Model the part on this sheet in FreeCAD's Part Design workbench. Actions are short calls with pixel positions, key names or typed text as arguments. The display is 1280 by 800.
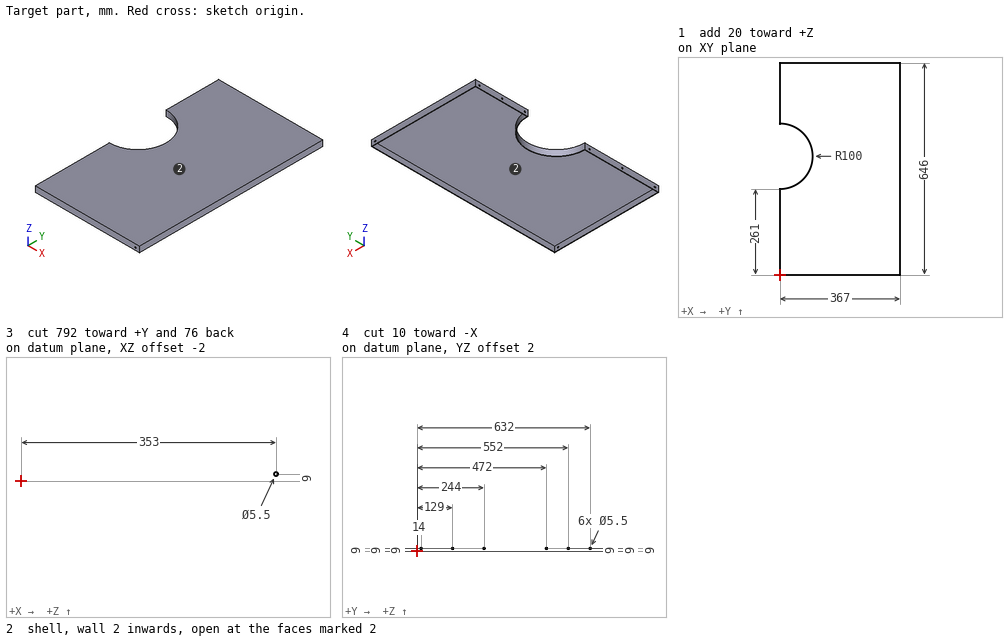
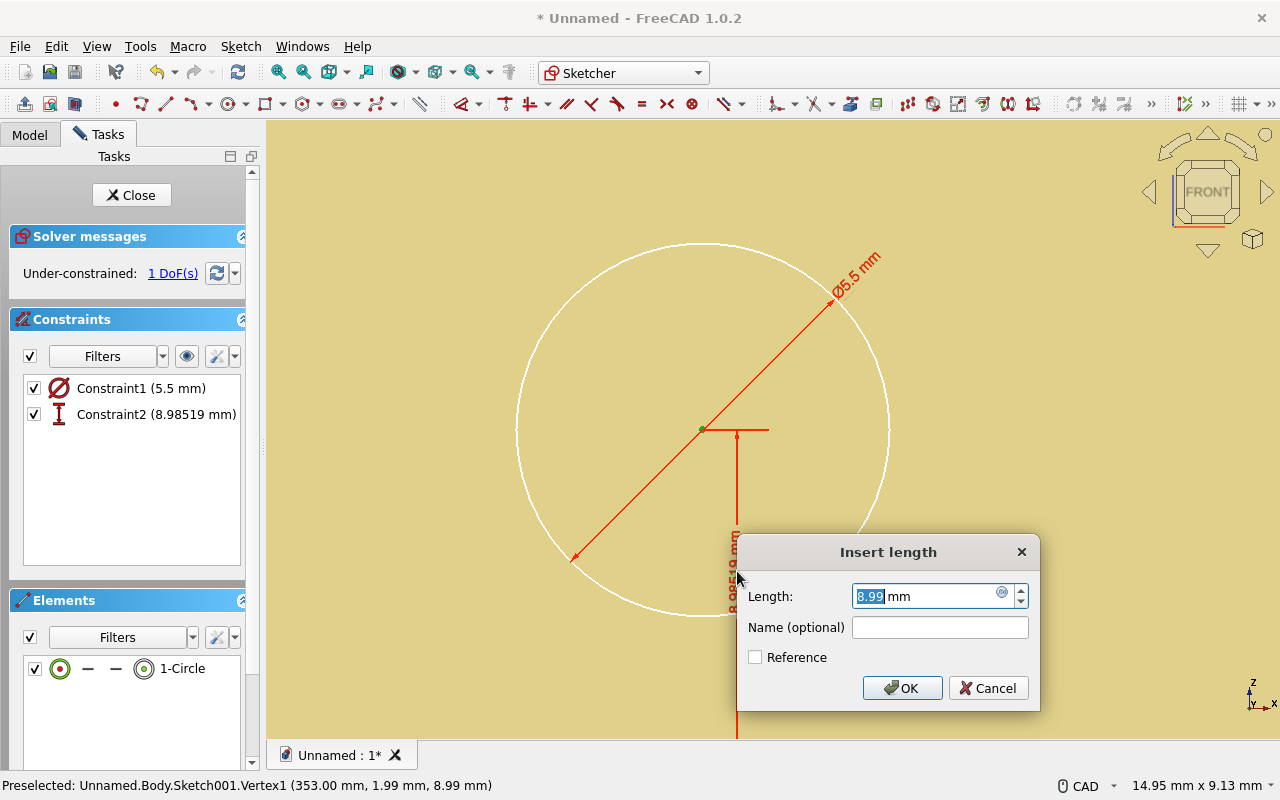
text(9)
key(Return)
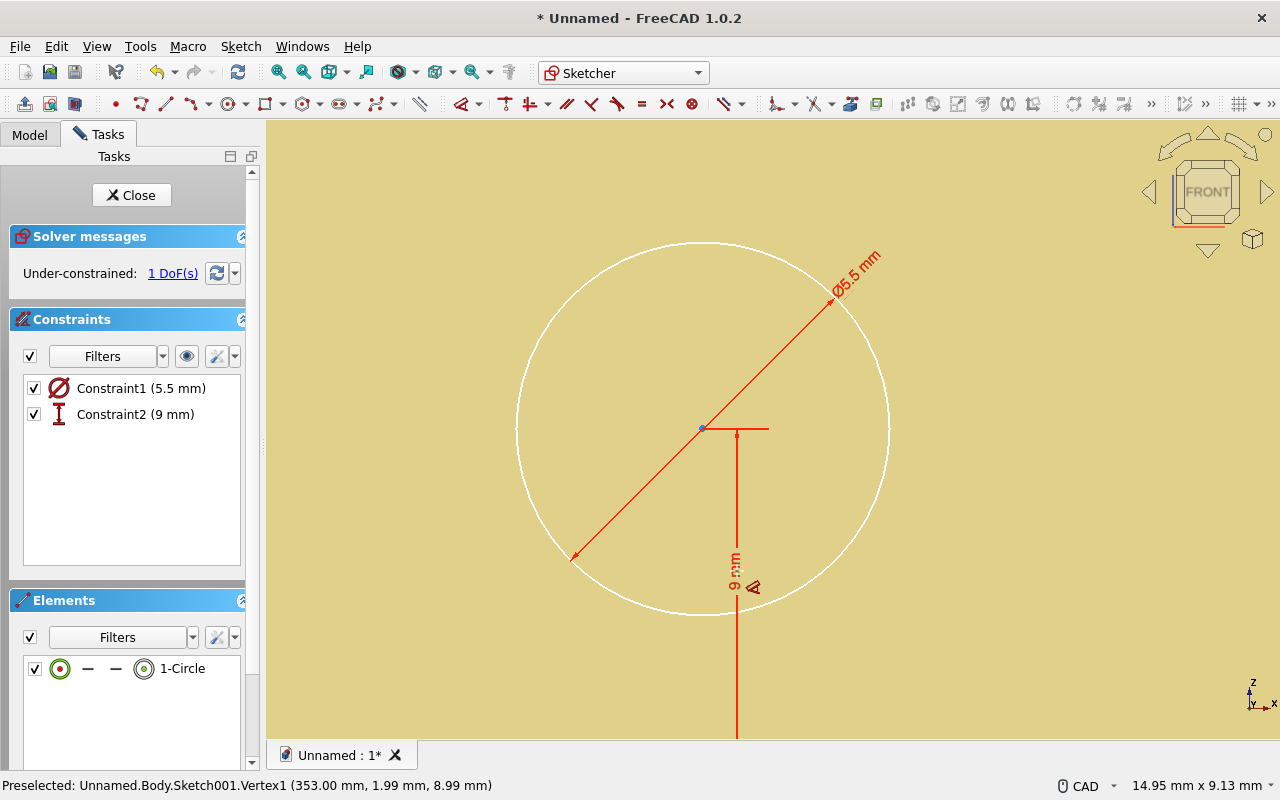
click(703, 429)
click(498, 395)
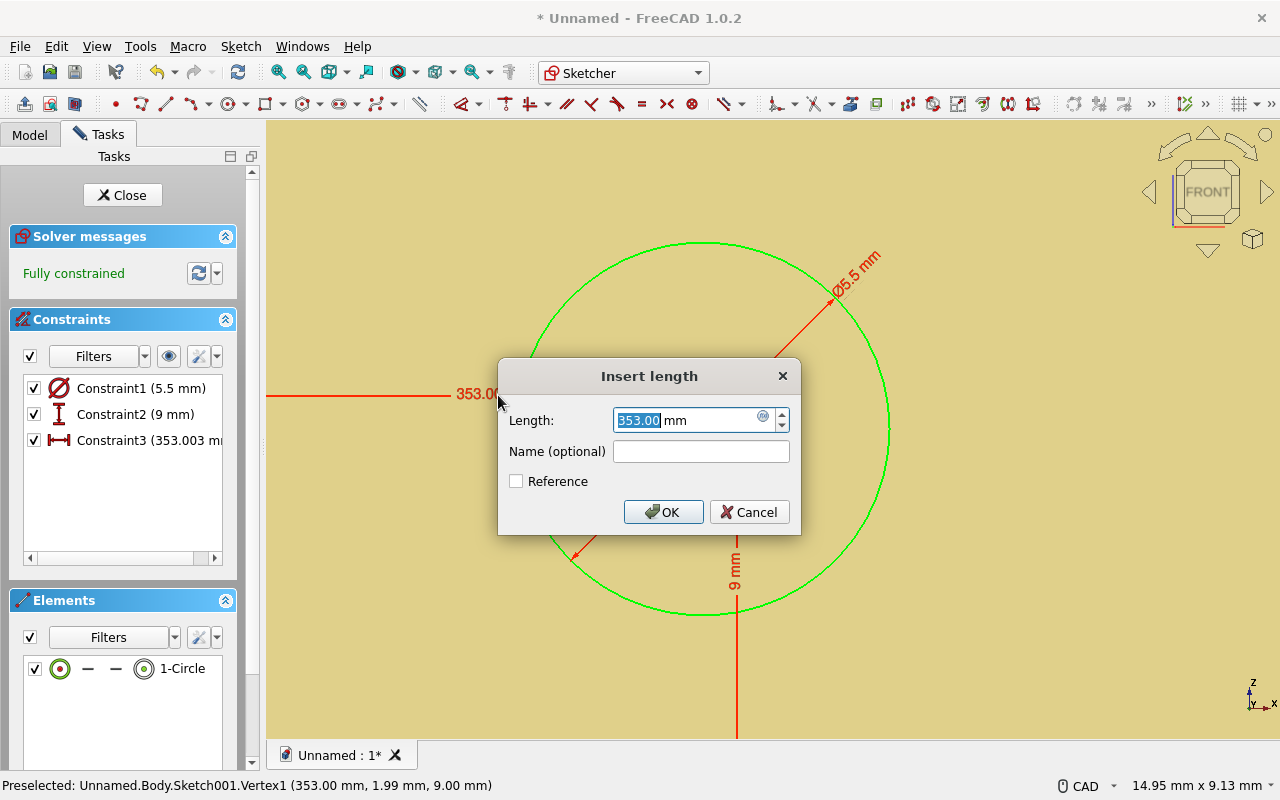
text(353)
key(Return)
key(Escape)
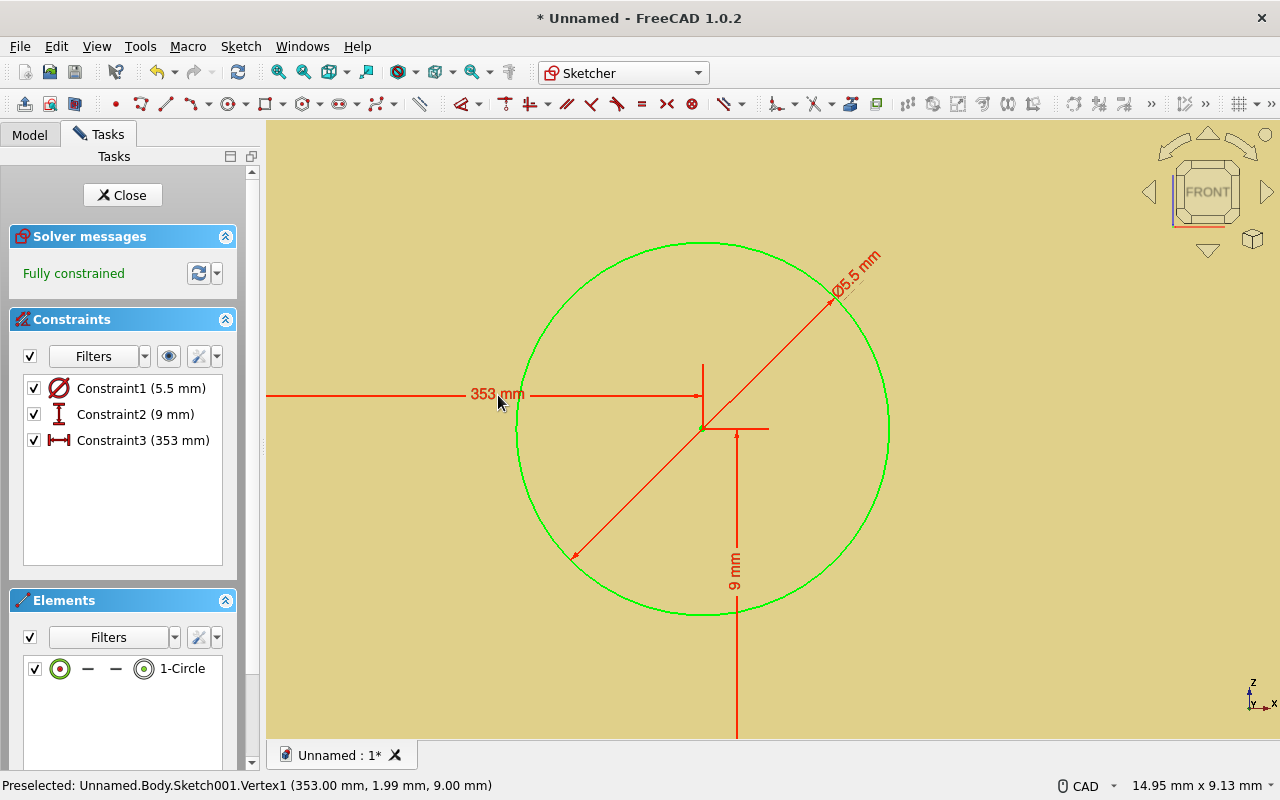
click(123, 195)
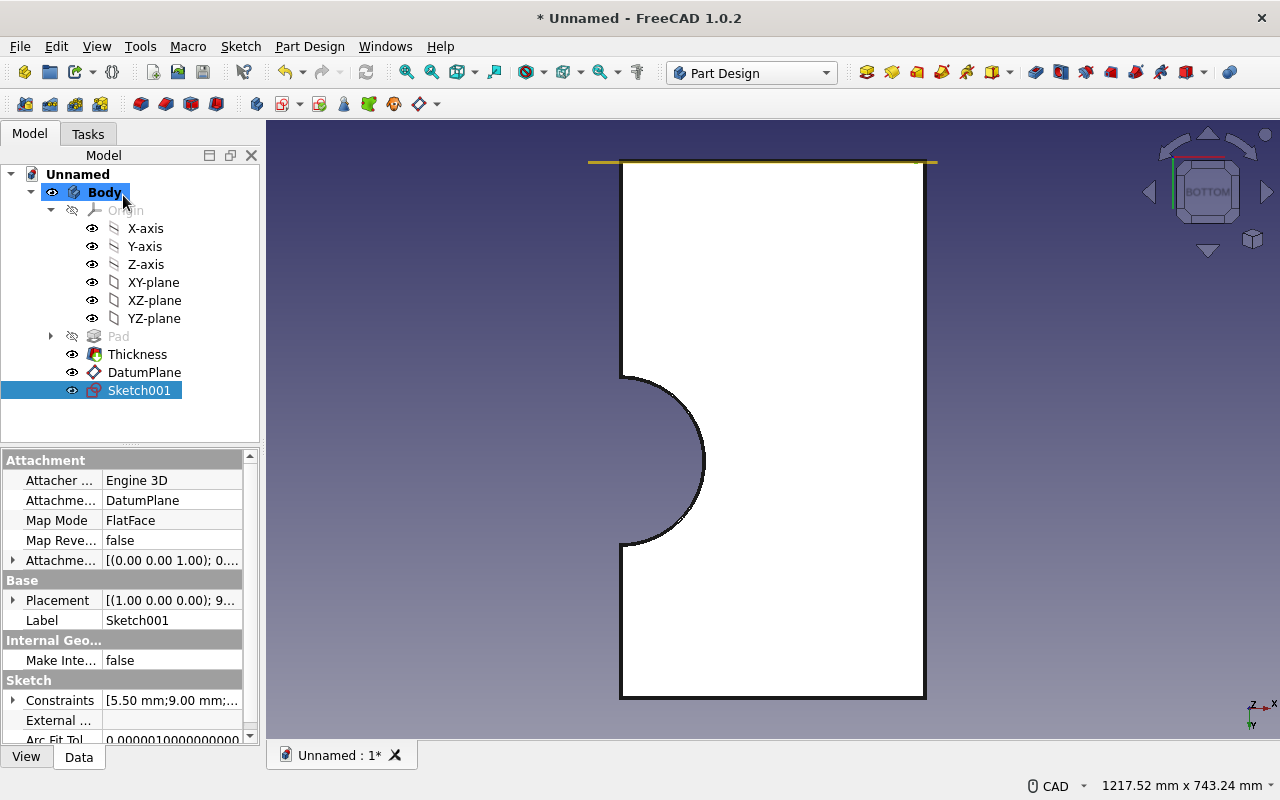
click(1036, 72)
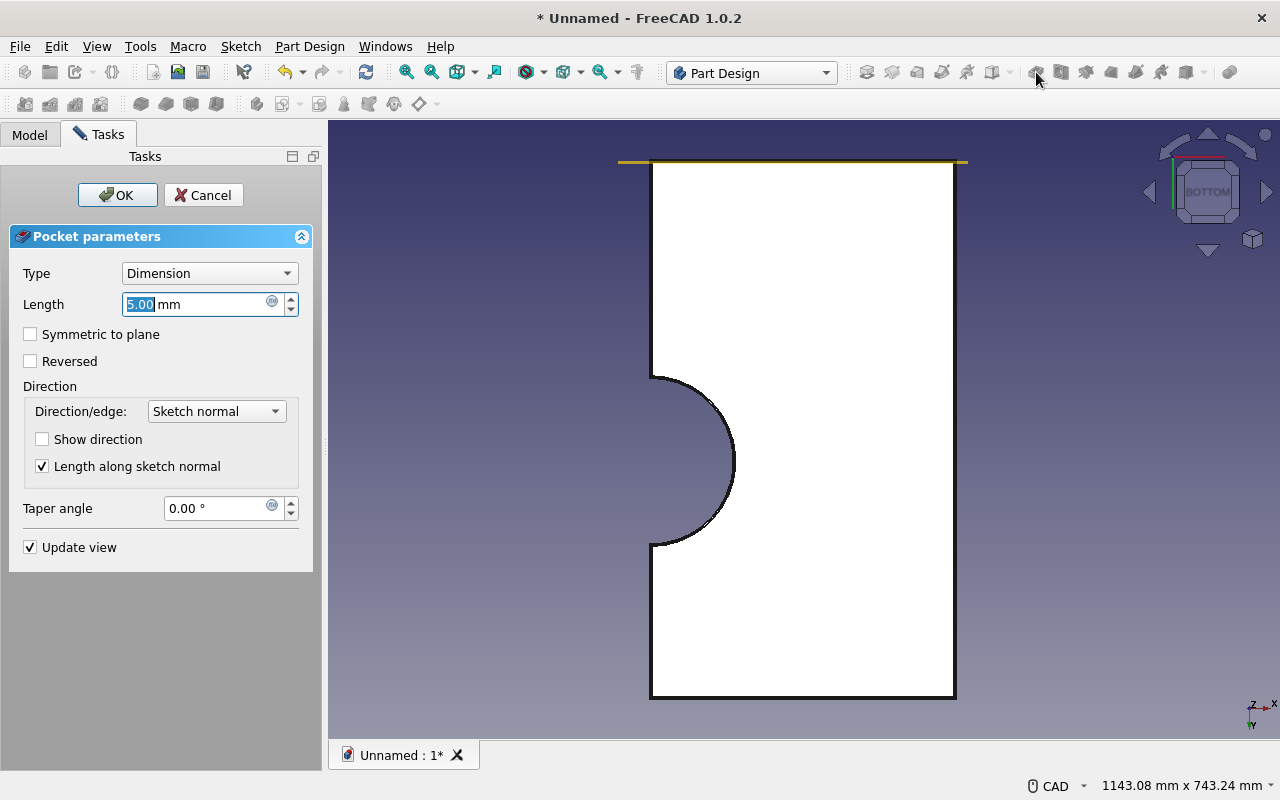
click(210, 274)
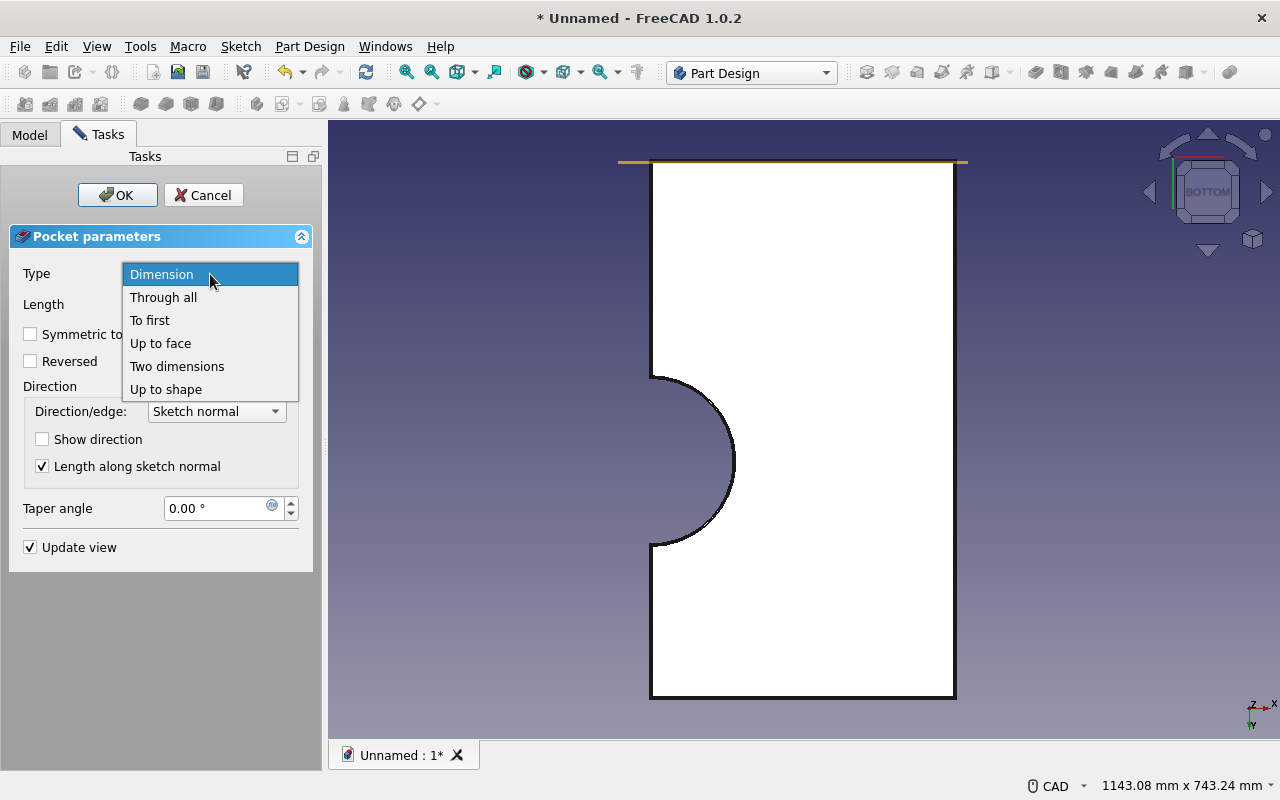
click(208, 366)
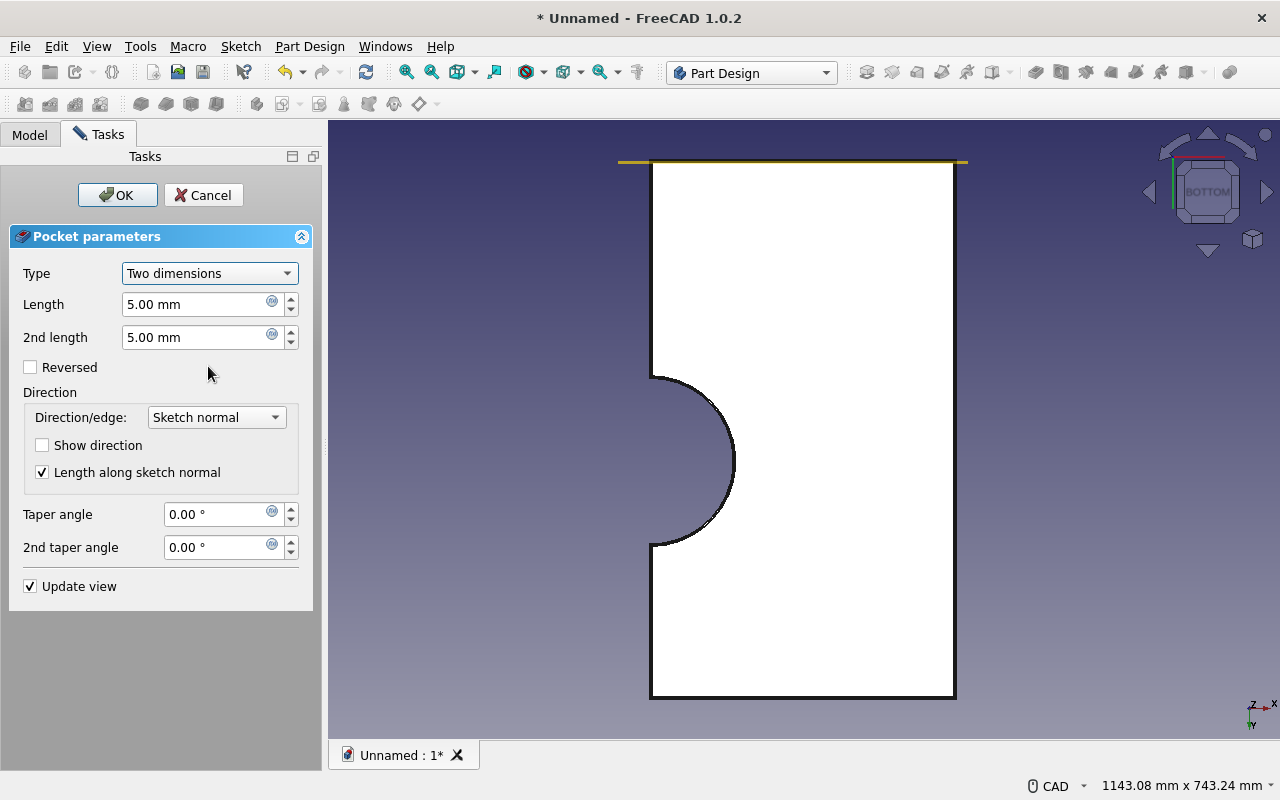
triple_click(204, 304)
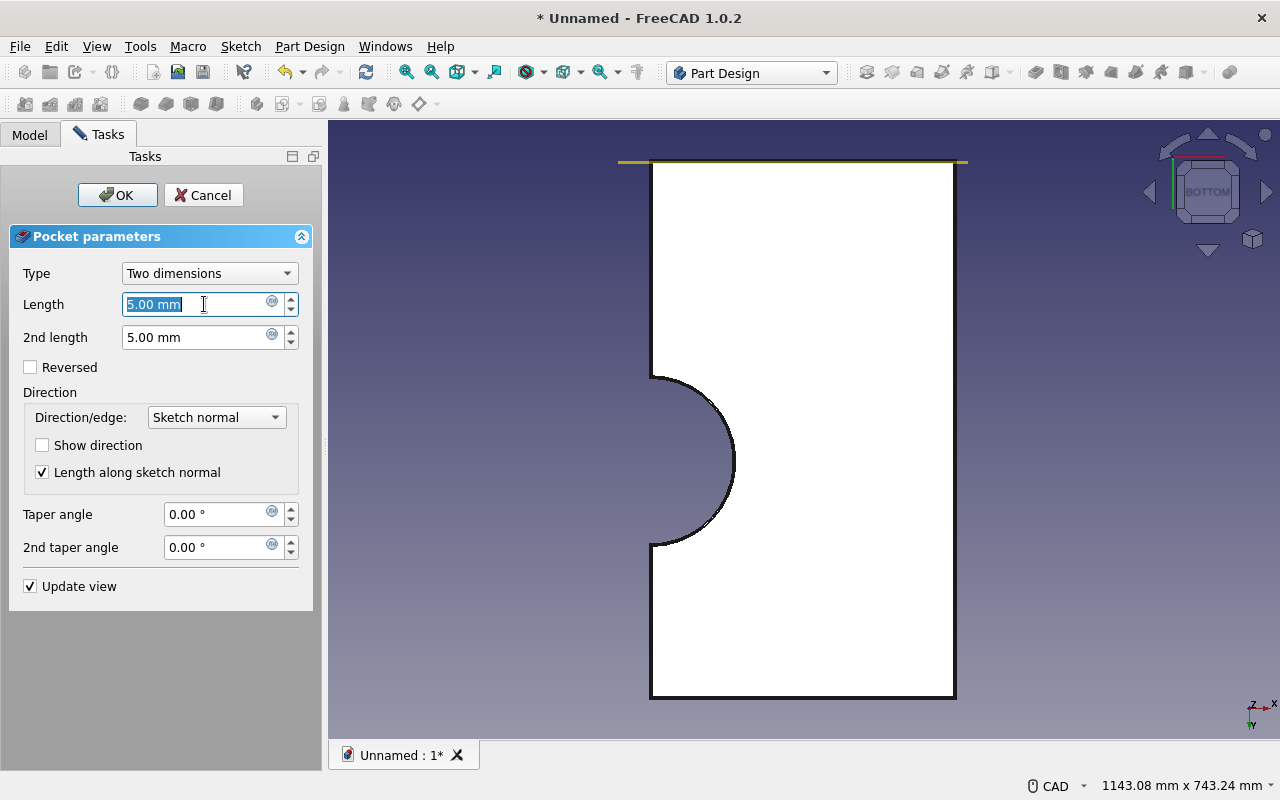
text(792)
key(Tab)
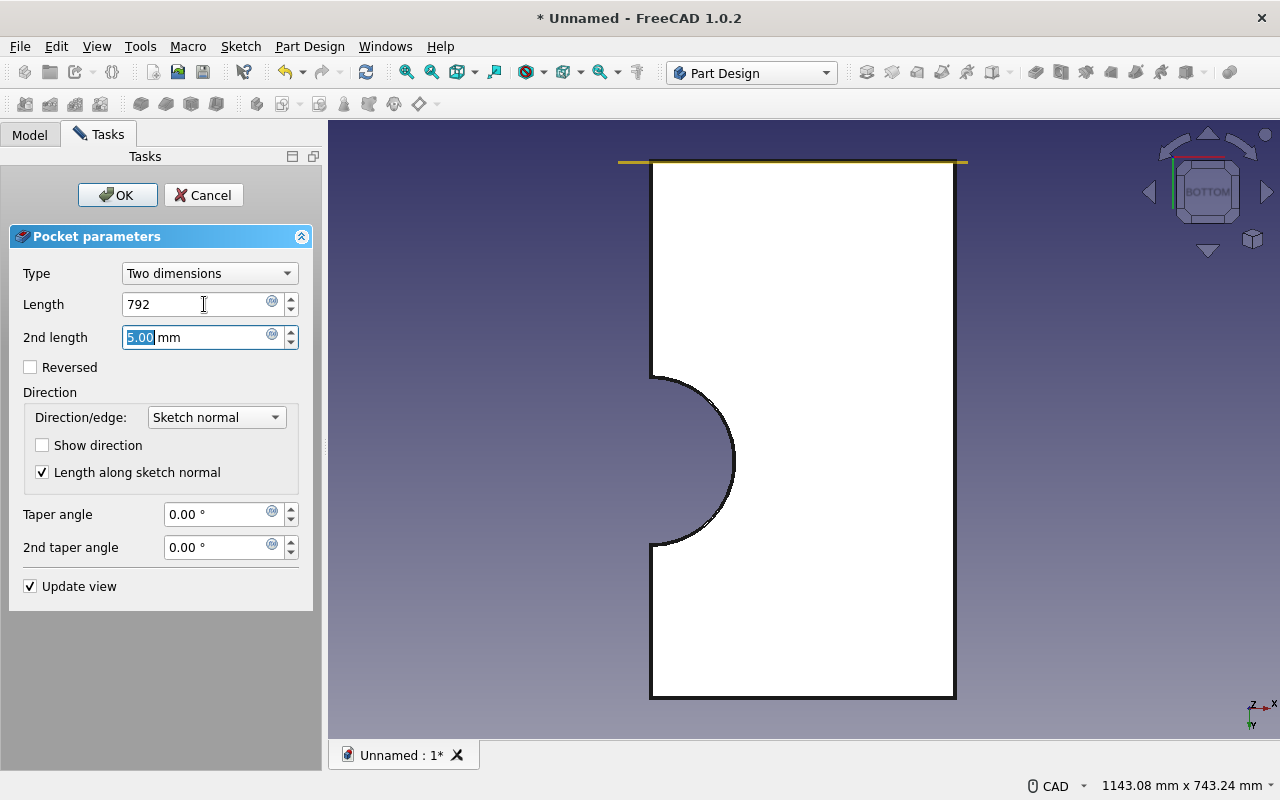
text(76)
key(Tab)